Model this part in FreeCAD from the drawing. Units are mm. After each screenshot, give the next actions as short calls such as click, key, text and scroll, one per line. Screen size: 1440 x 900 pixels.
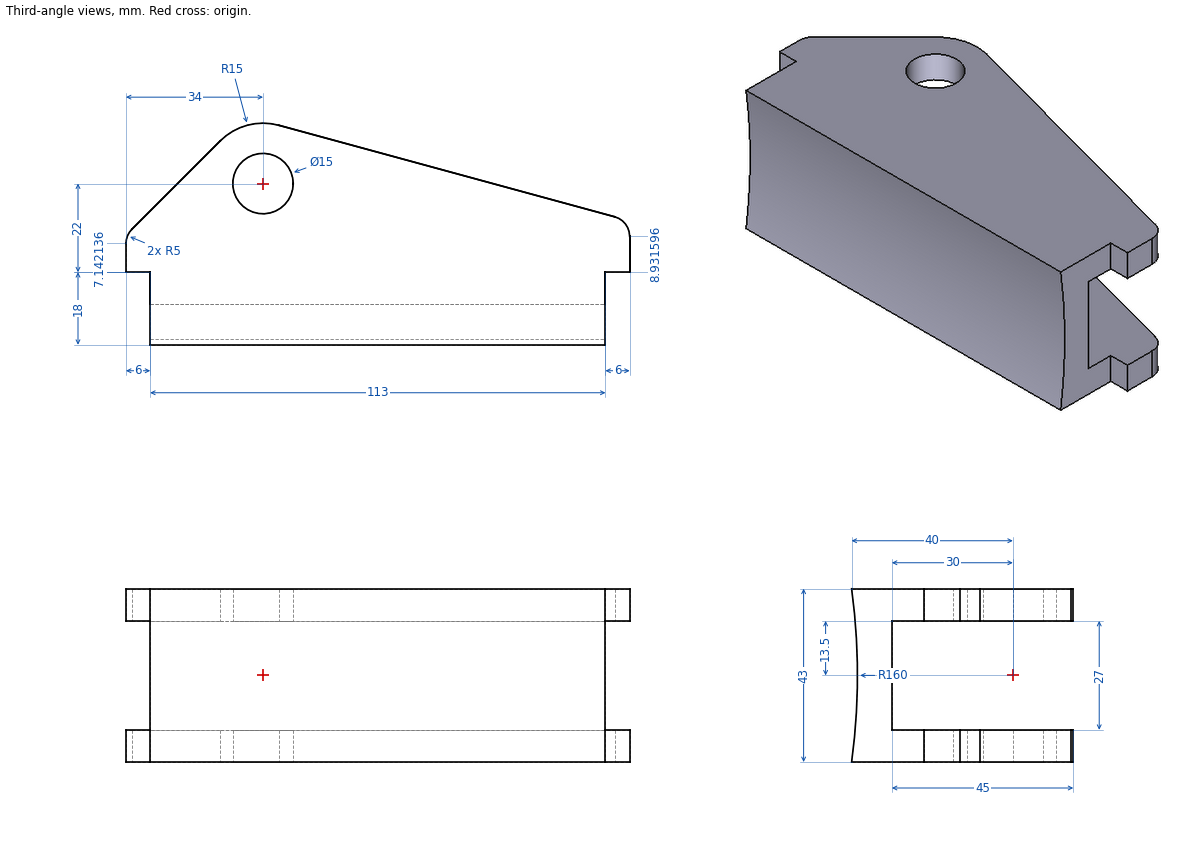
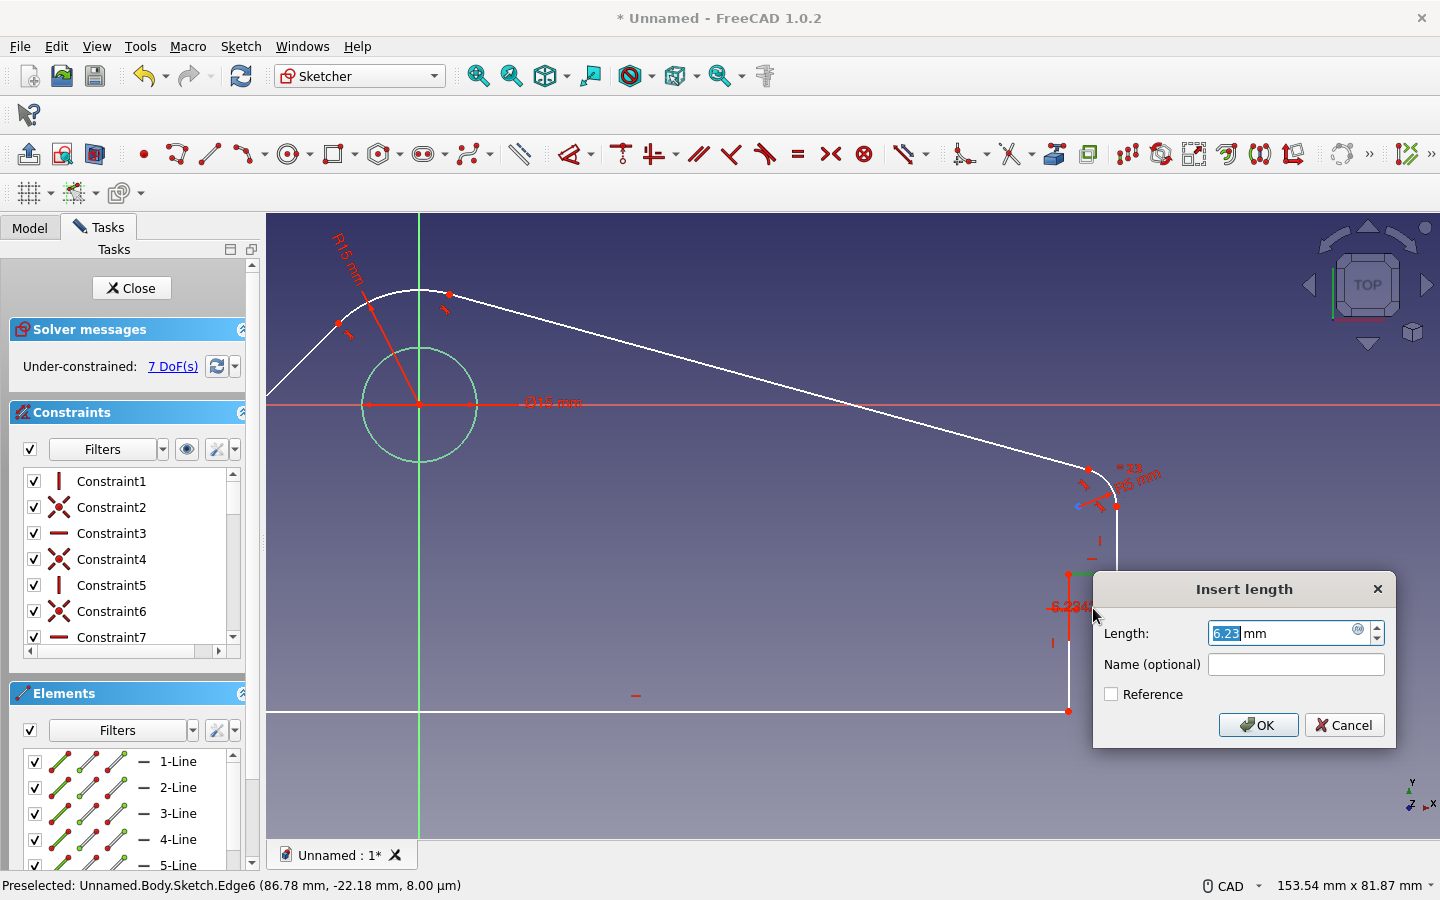
text(6)
key(Return)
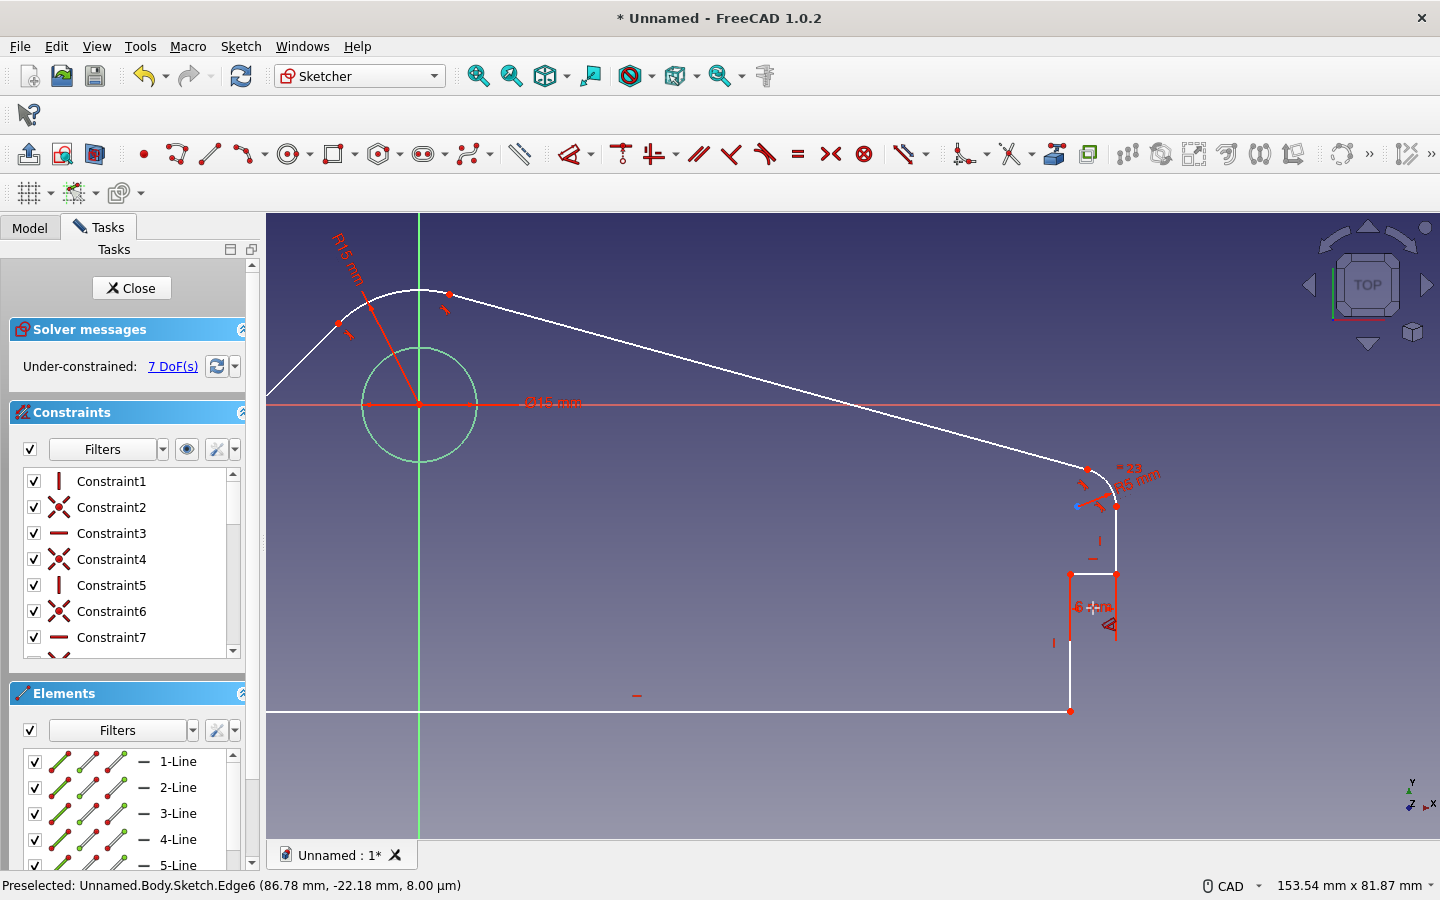
scroll(1084, 574, down, 2)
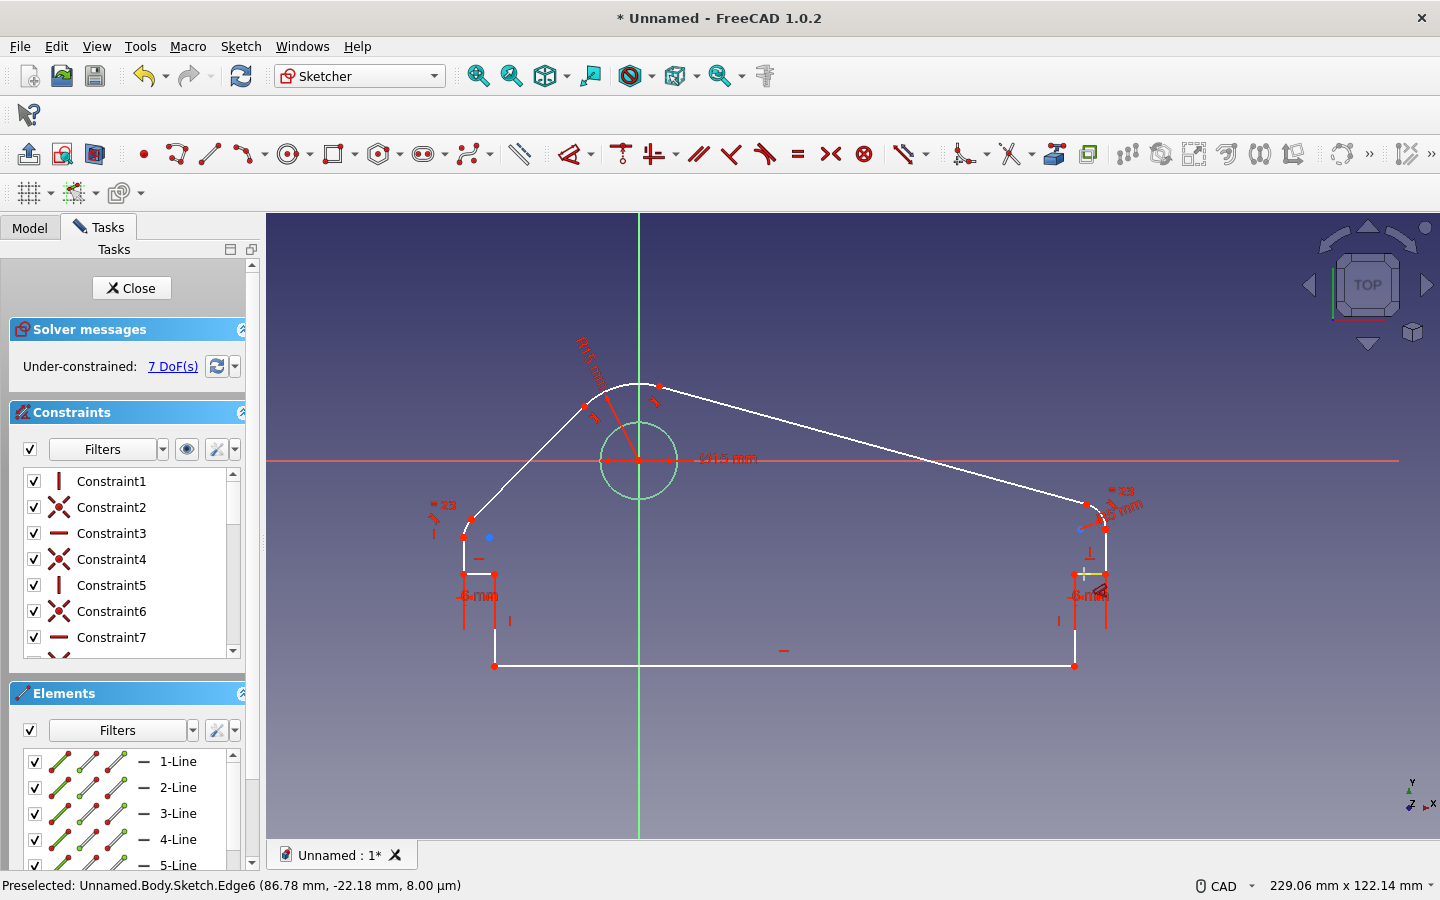
click(495, 602)
click(461, 620)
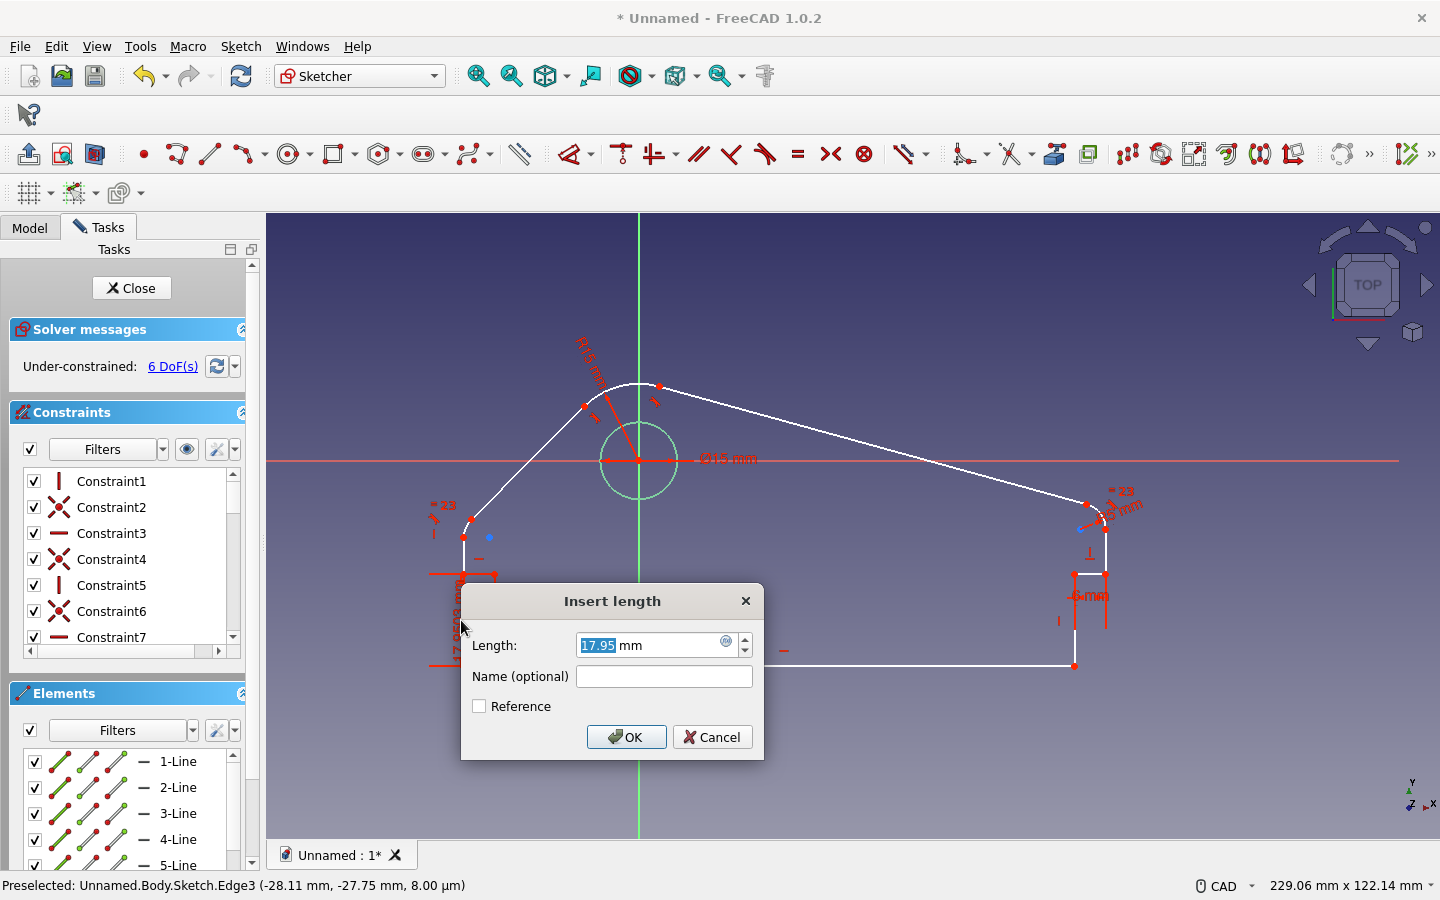
text(18)
key(Return)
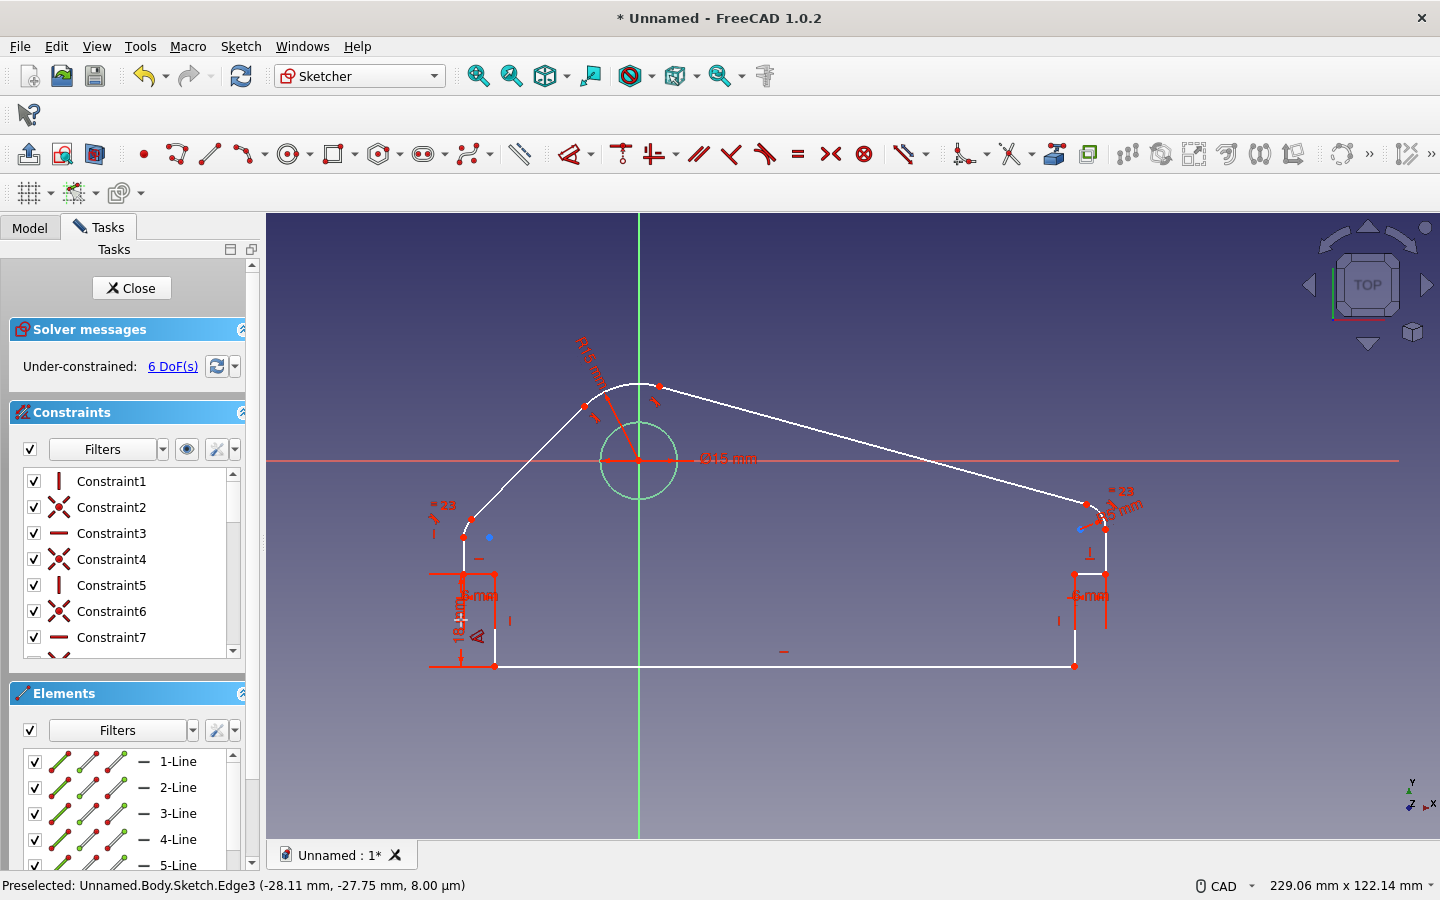
click(1075, 639)
click(1109, 621)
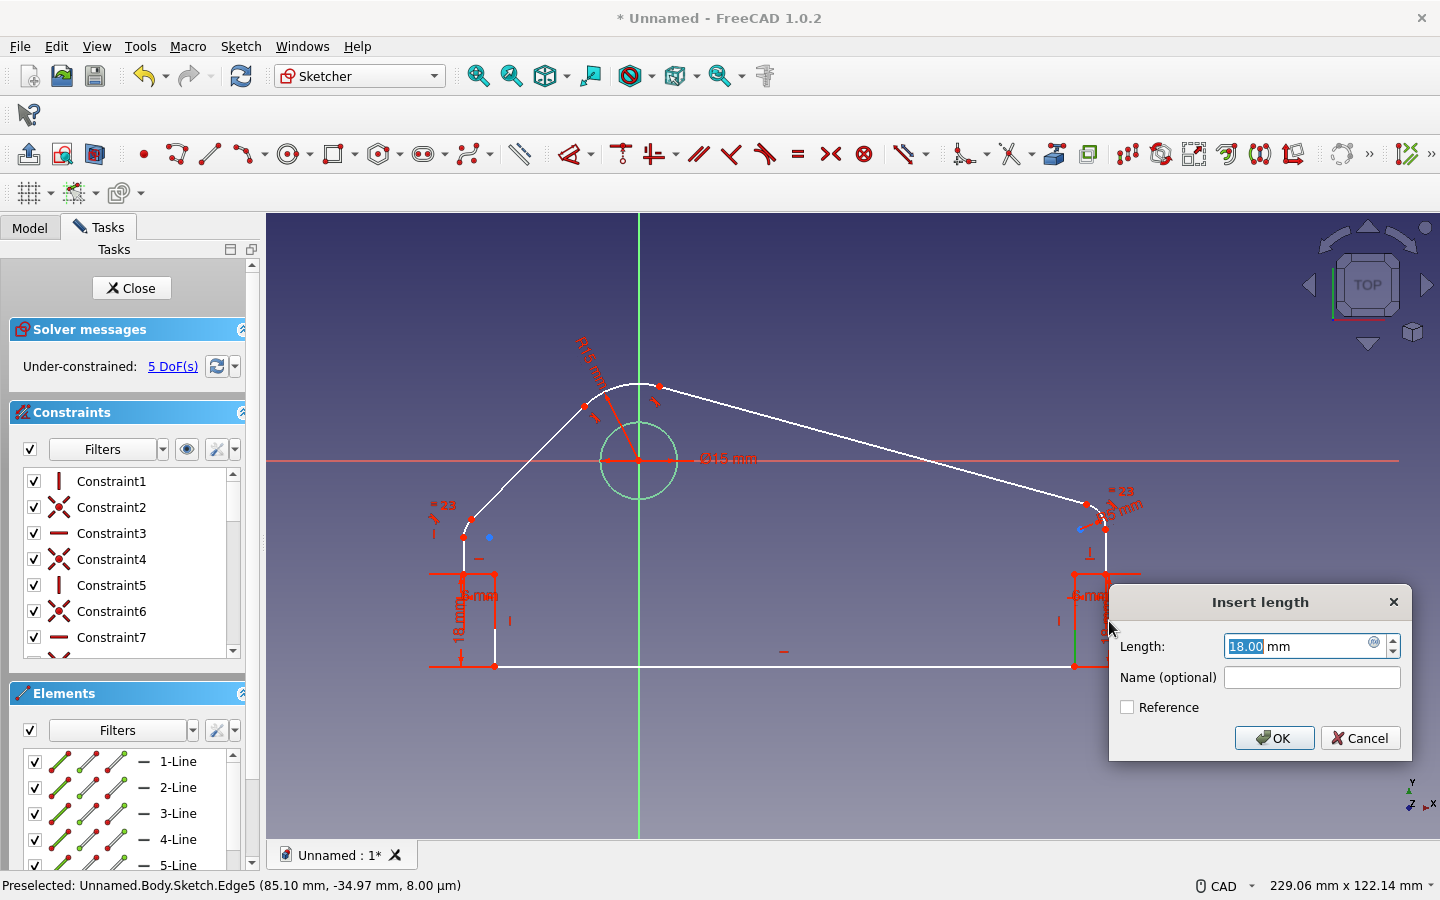
text(18)
key(Return)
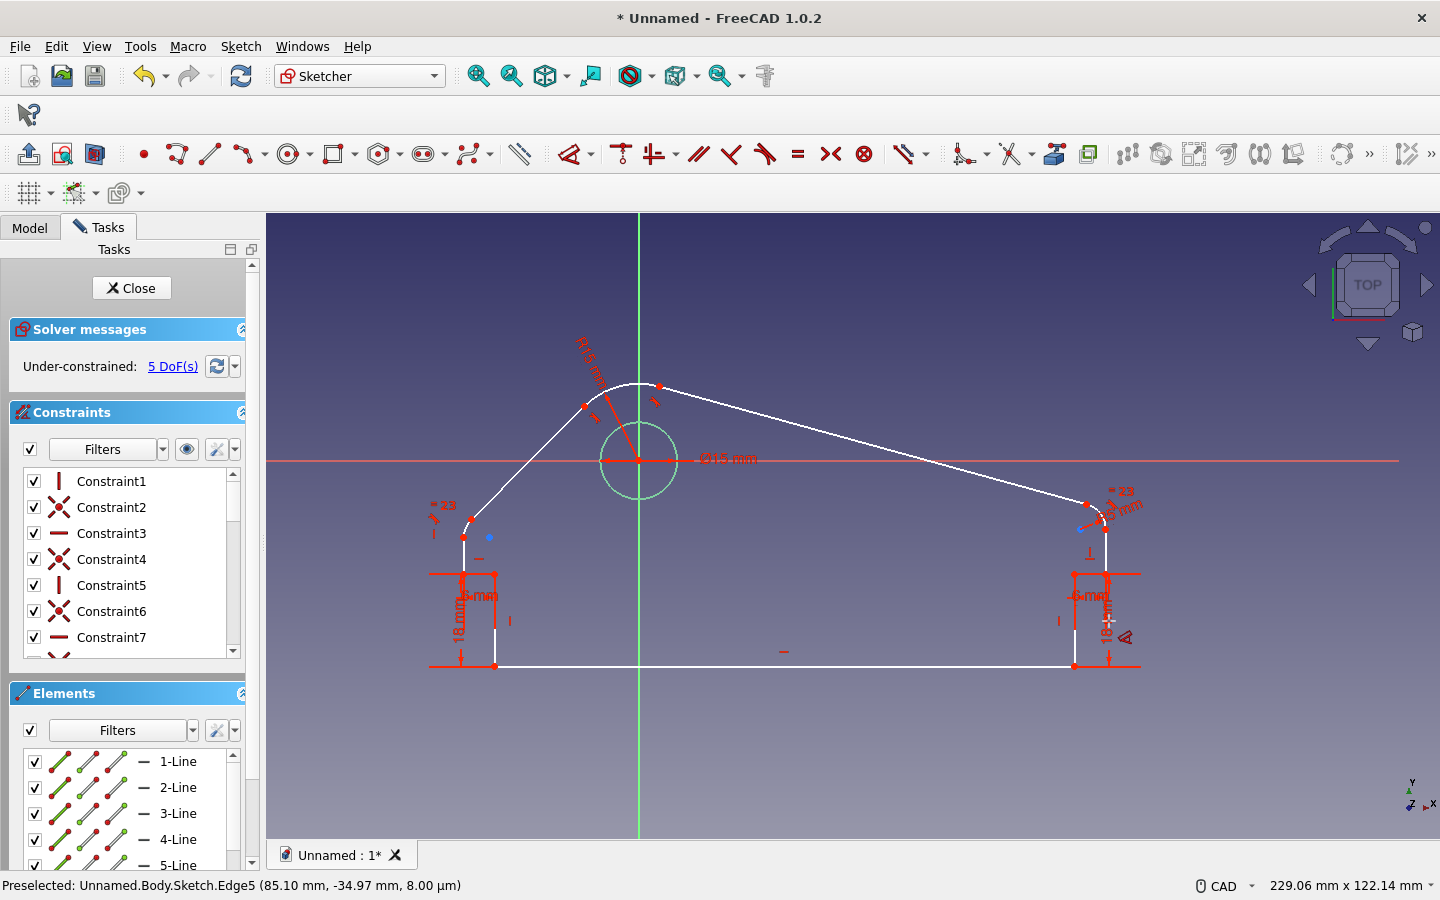
click(669, 667)
click(785, 701)